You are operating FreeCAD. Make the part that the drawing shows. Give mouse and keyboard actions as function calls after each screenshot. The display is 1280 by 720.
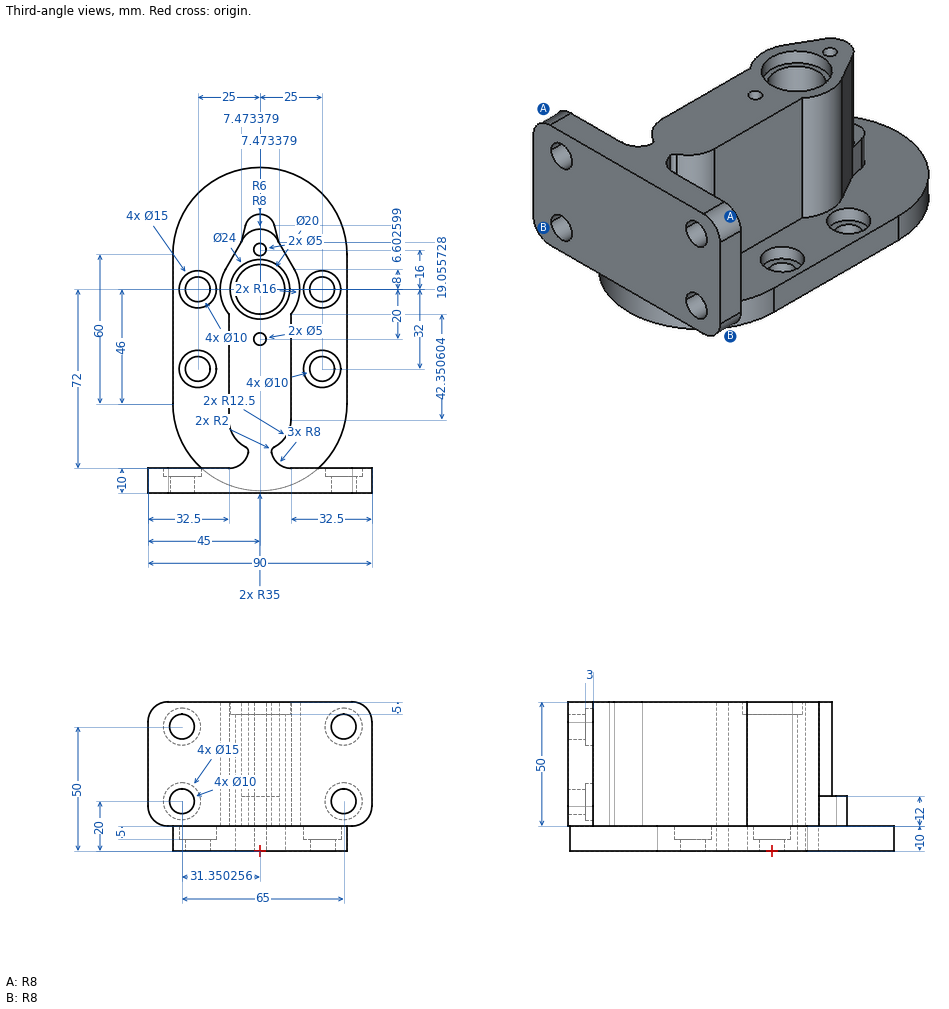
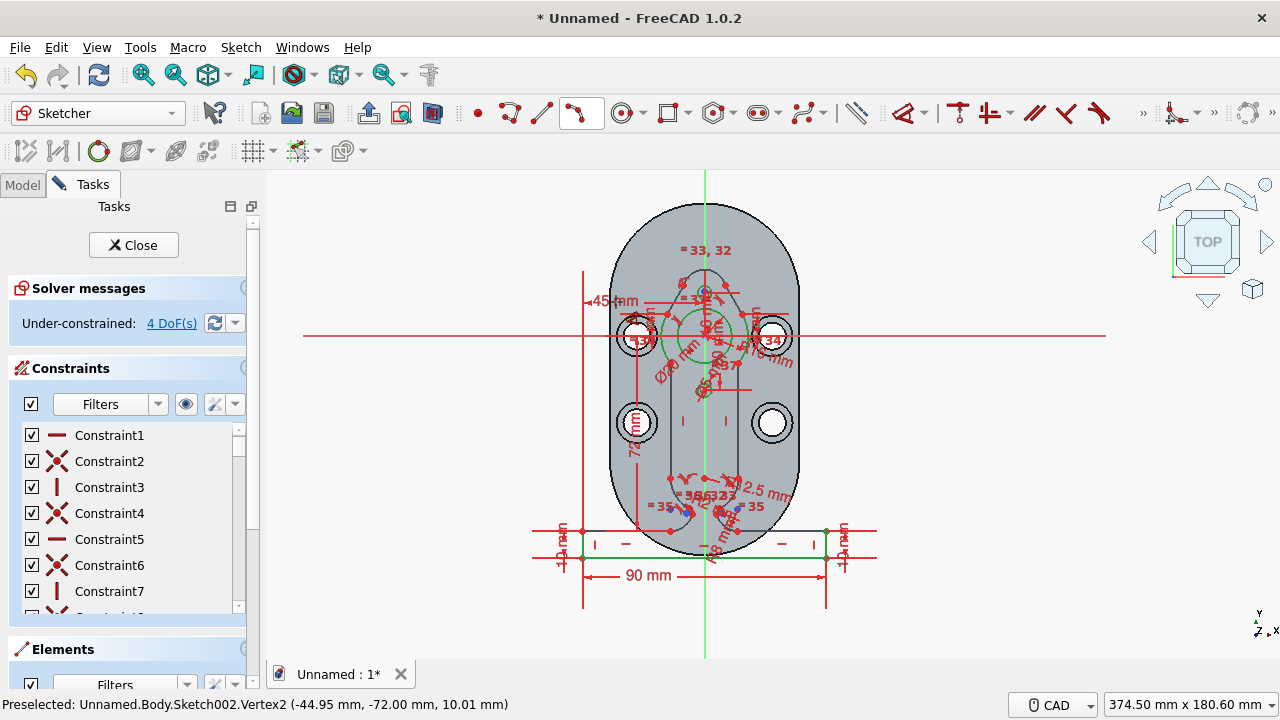
click(645, 531)
click(627, 497)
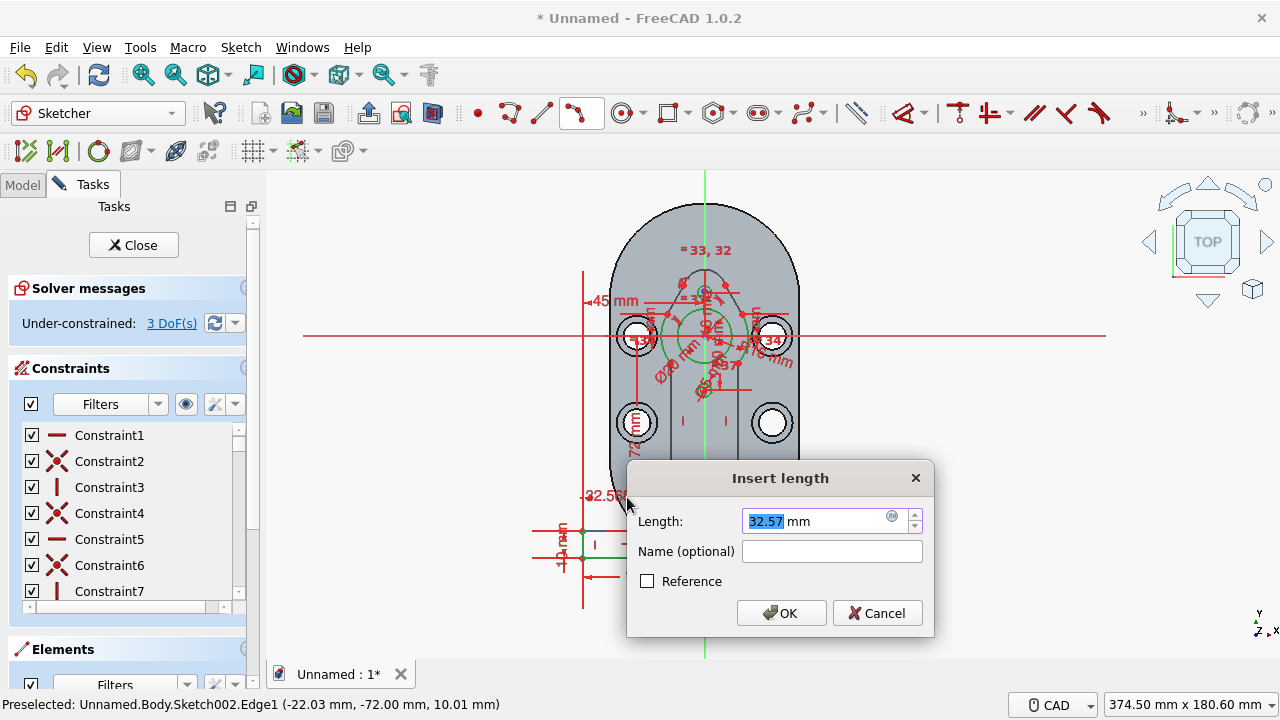
text(32.5)
key(Return)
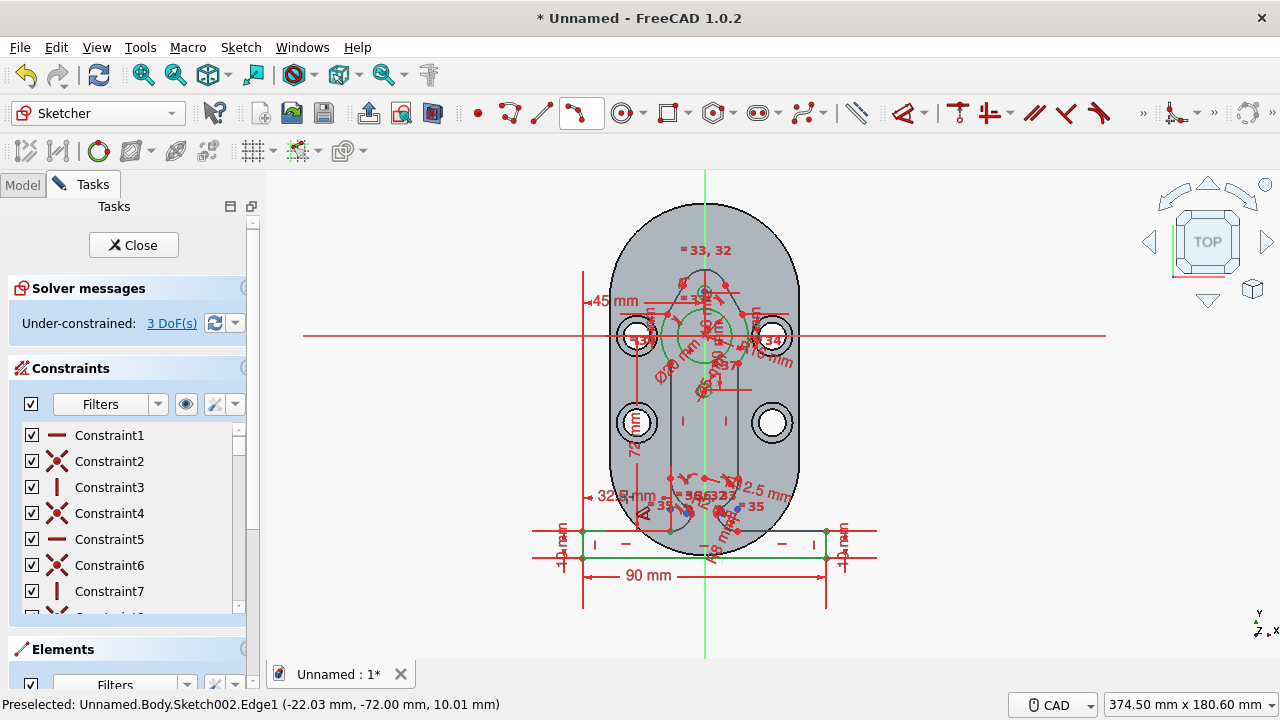
click(800, 531)
click(782, 589)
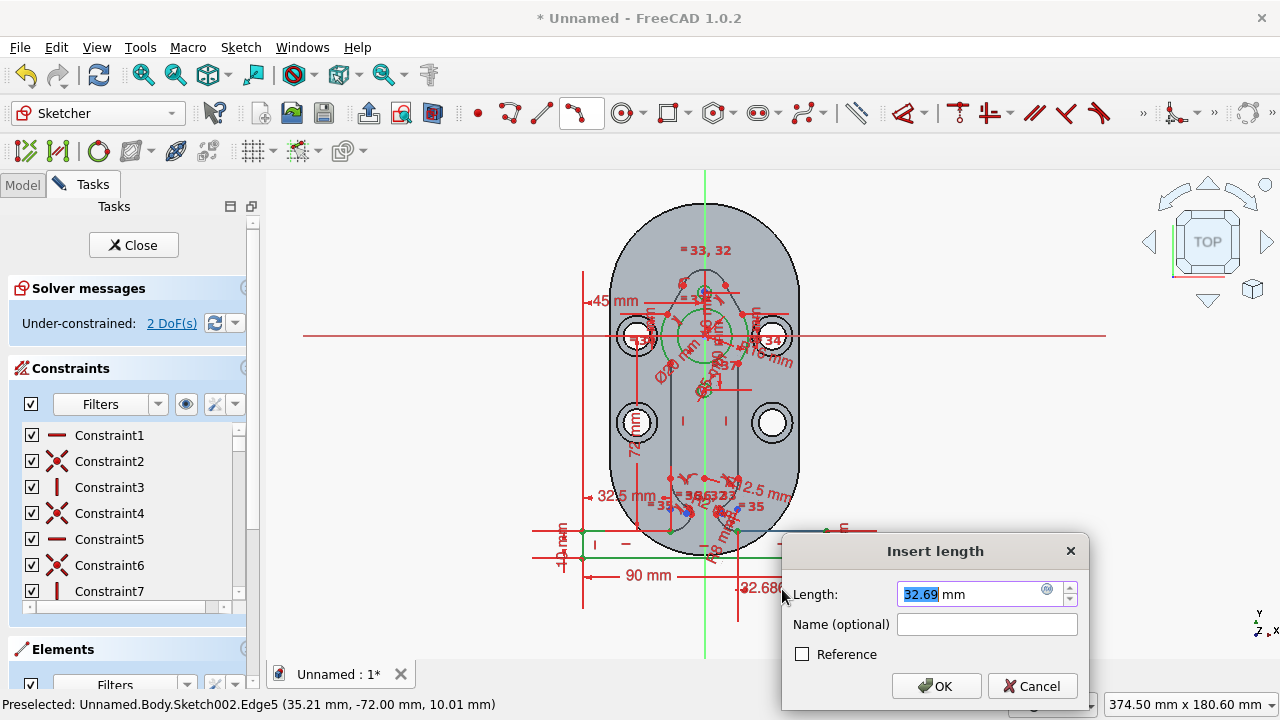
text(32.5)
key(Return)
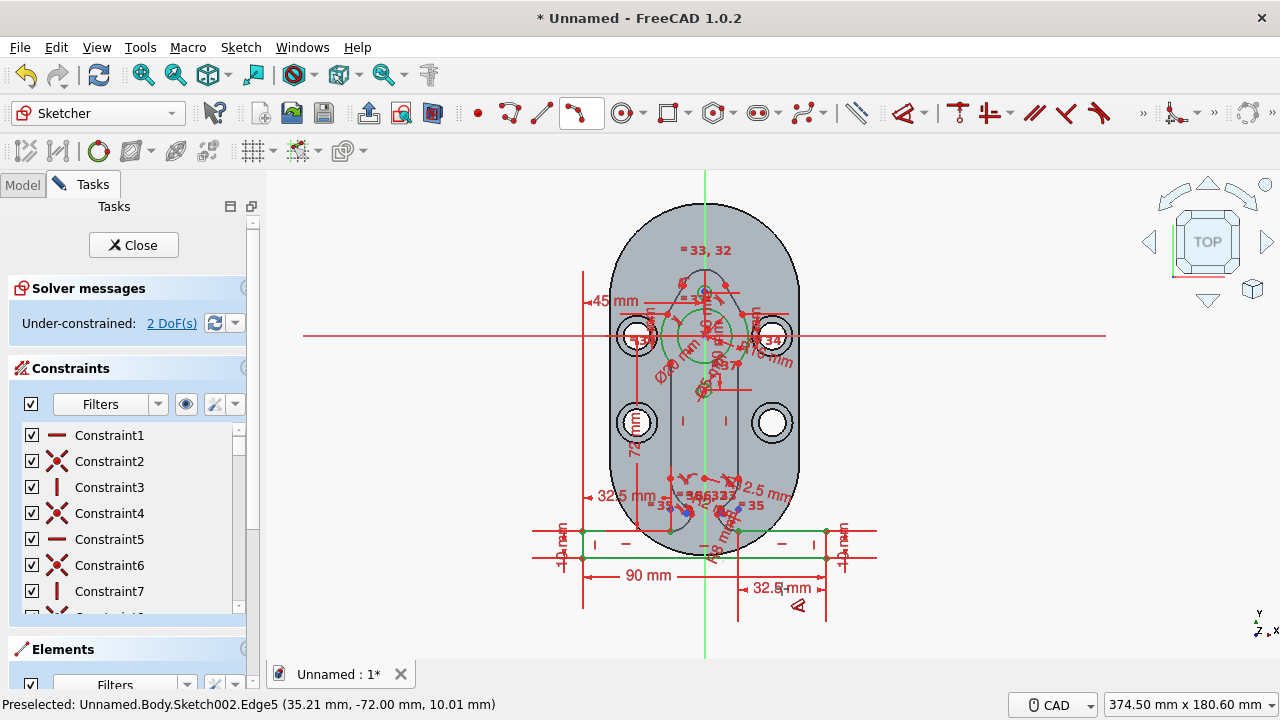
click(738, 444)
click(772, 421)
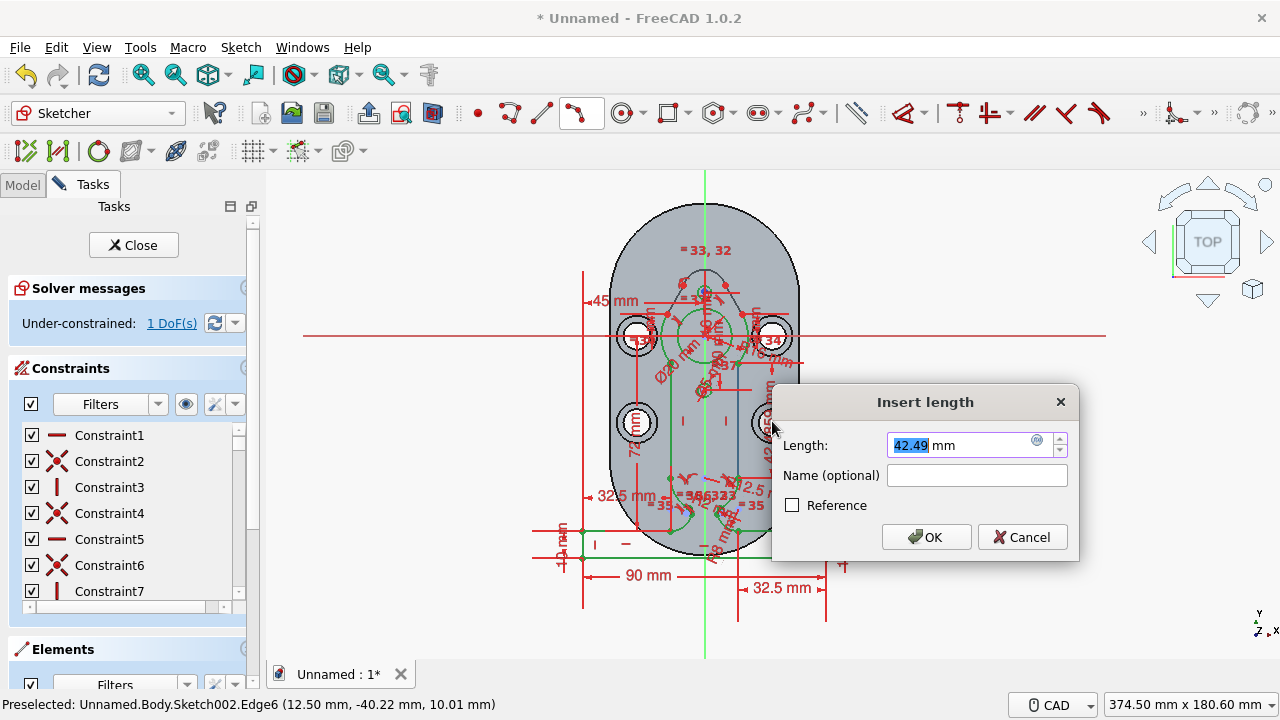
text(42.350604)
key(Return)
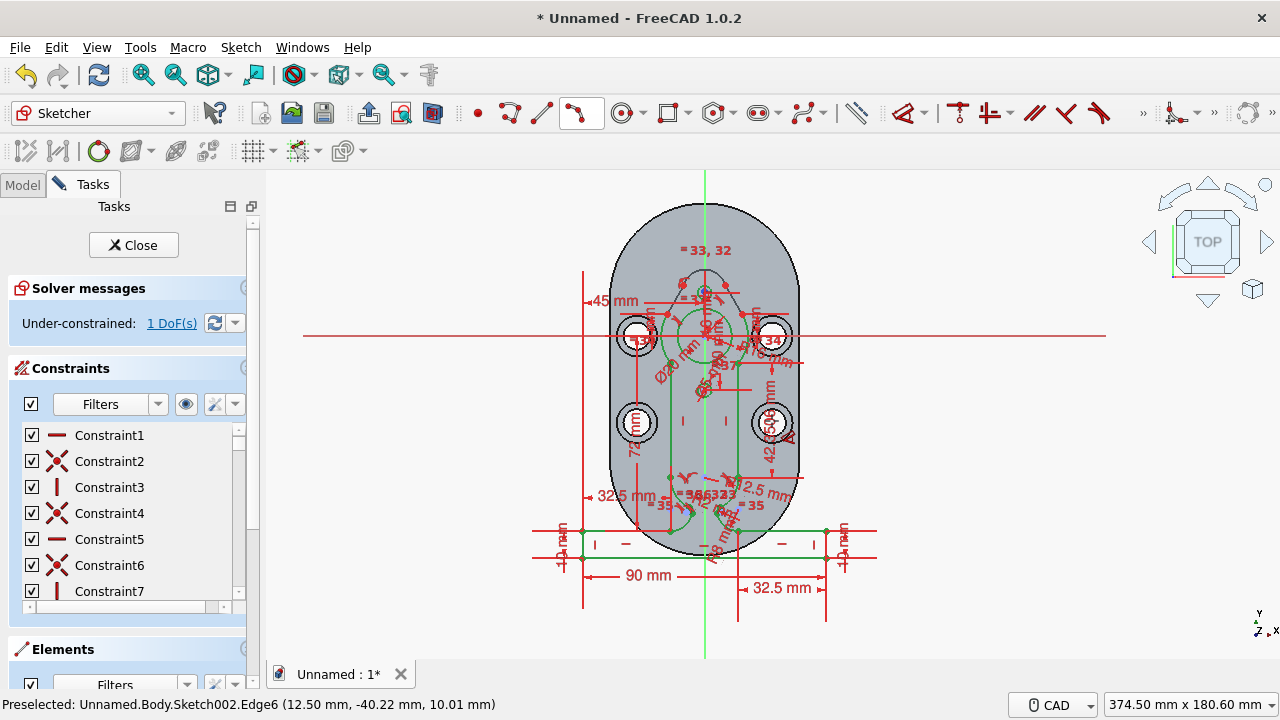
scroll(726, 286, up, 4)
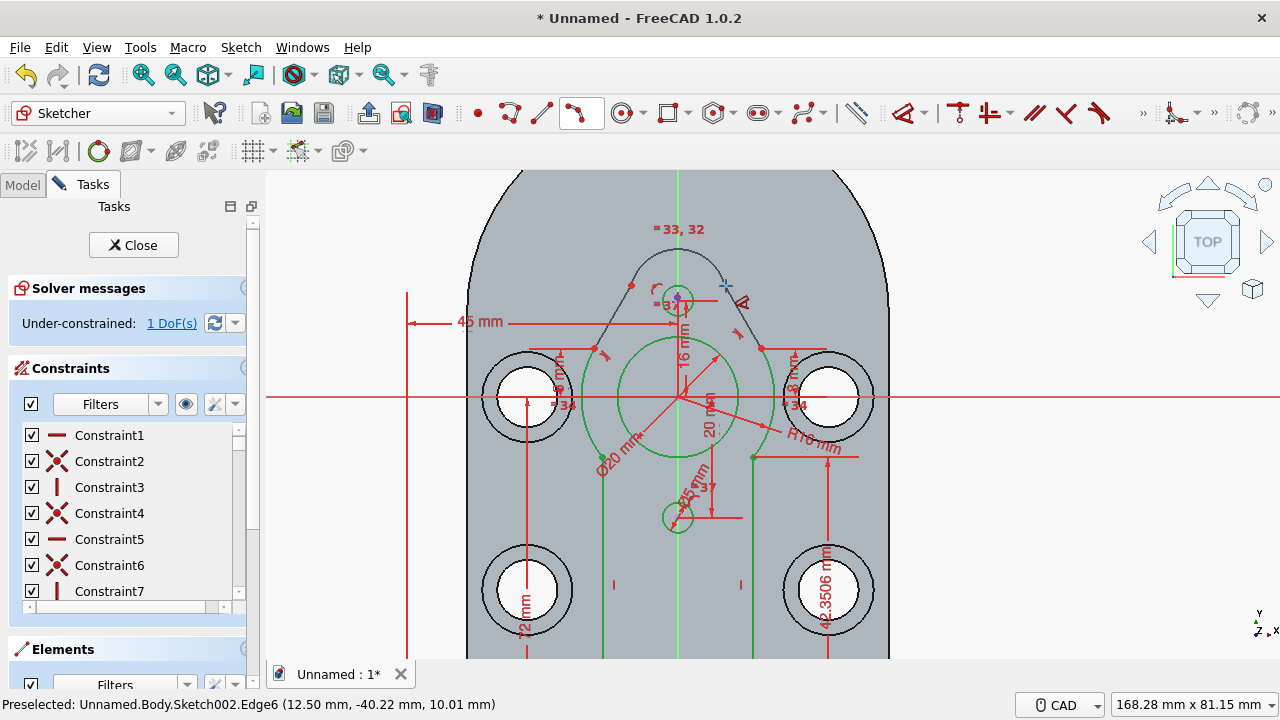
click(725, 285)
click(701, 227)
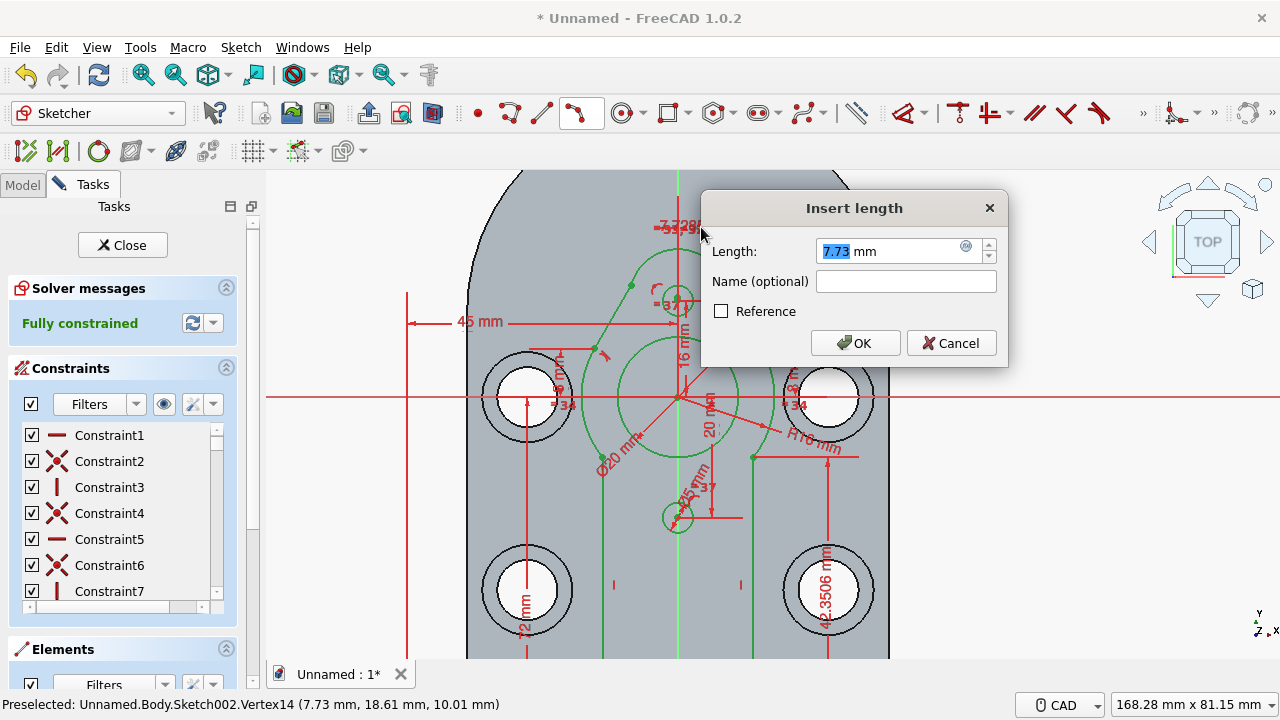
text(7.473379)
key(Return)
key(Escape)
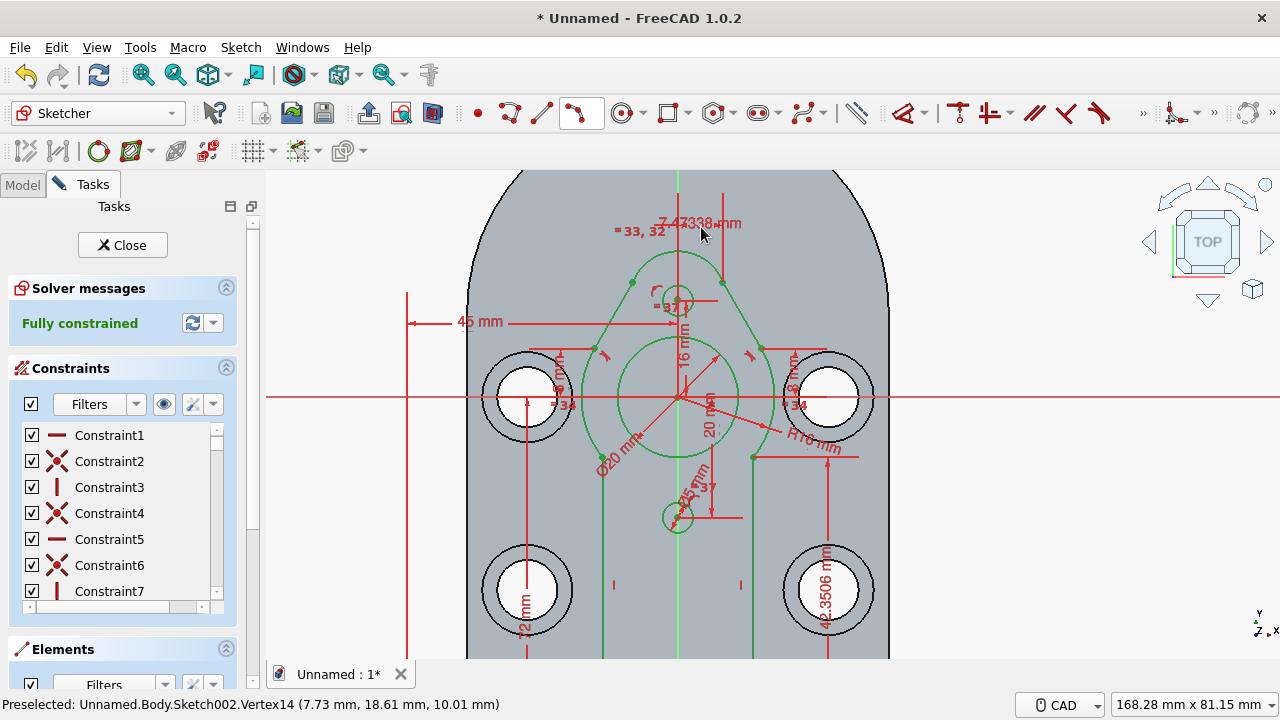
click(123, 245)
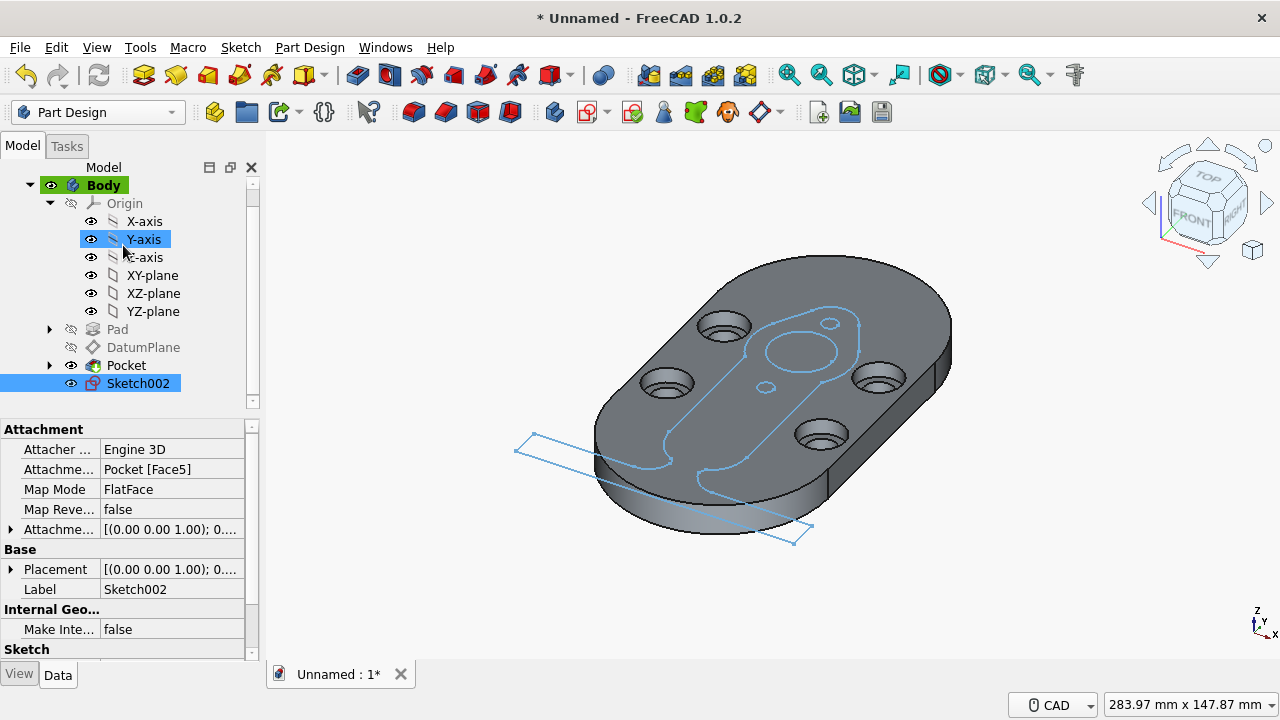
click(144, 76)